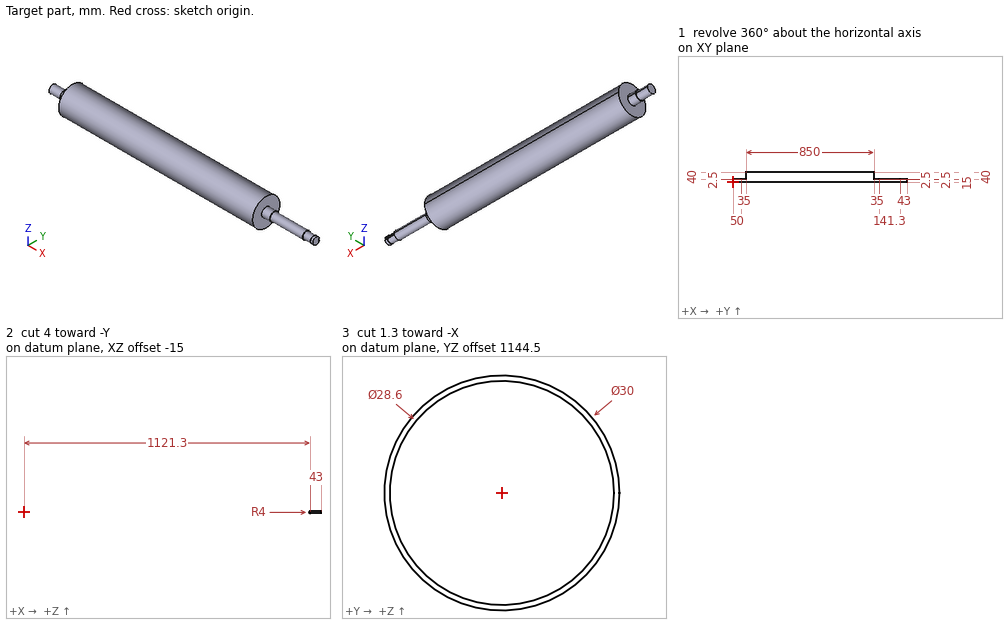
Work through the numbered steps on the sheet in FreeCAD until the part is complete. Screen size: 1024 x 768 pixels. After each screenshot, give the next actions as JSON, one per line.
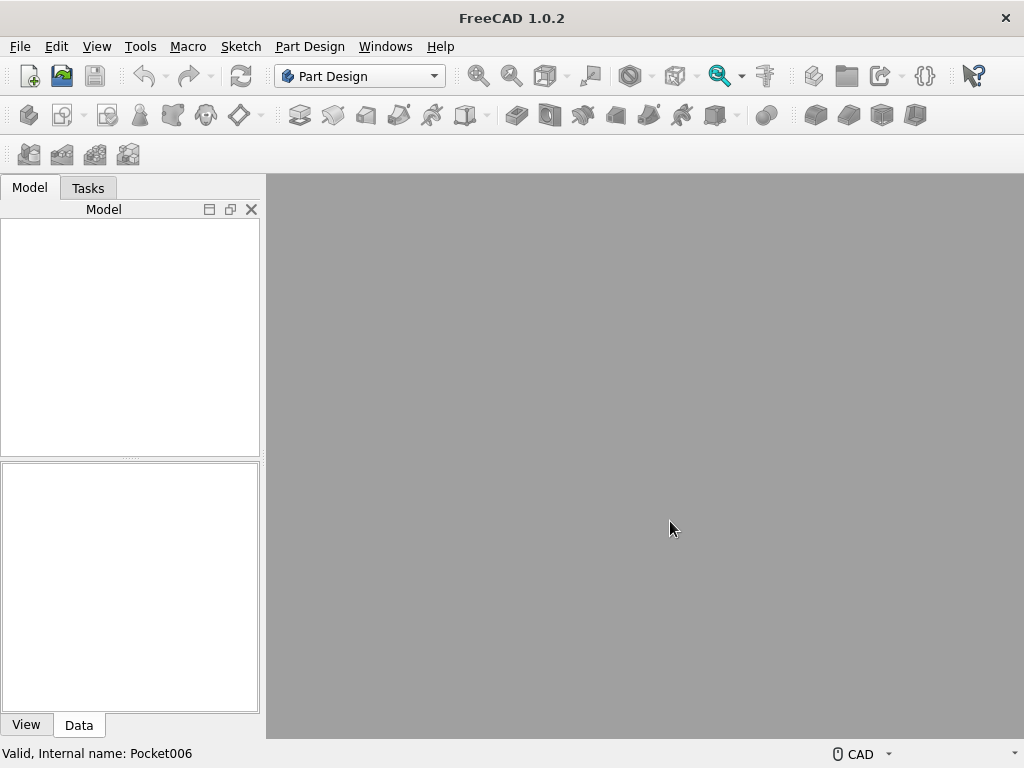
{"action": "key", "text": "ctrl+n"}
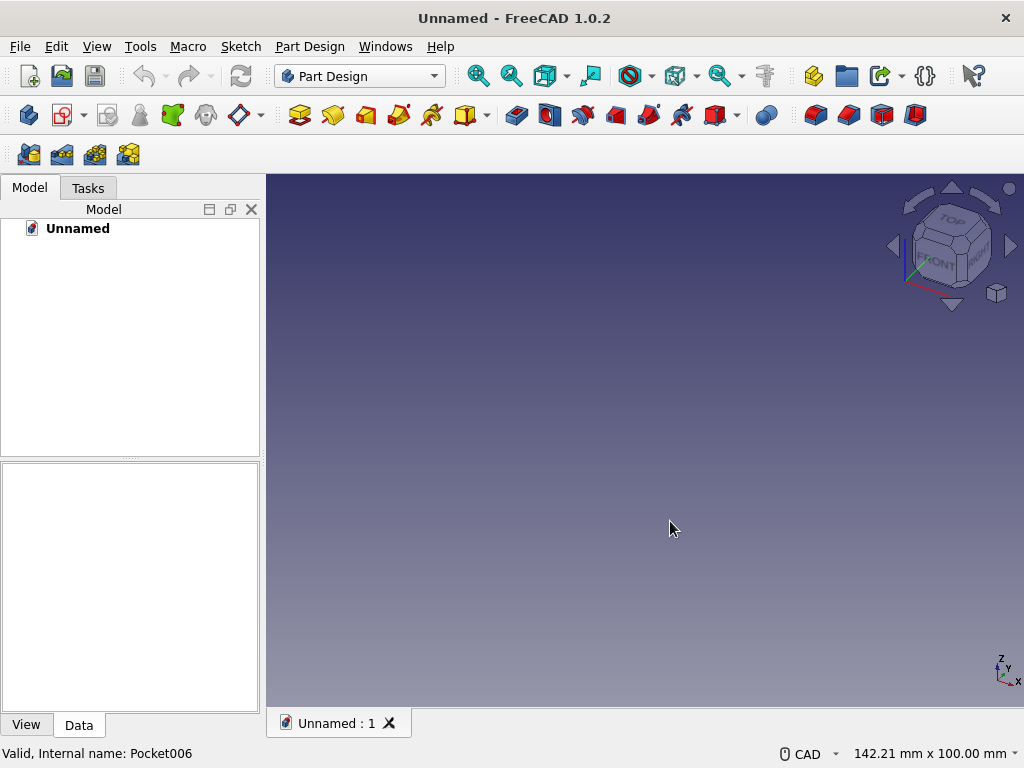
{"action": "left_click", "coordinate": [62, 116]}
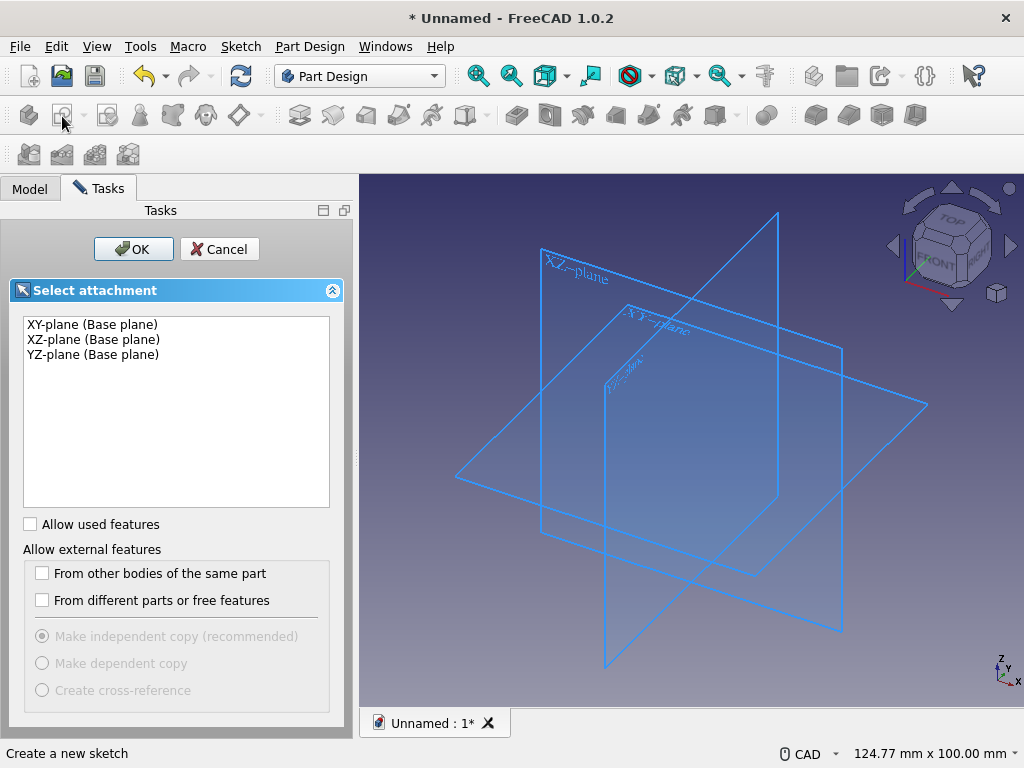
{"action": "left_click", "coordinate": [84, 324]}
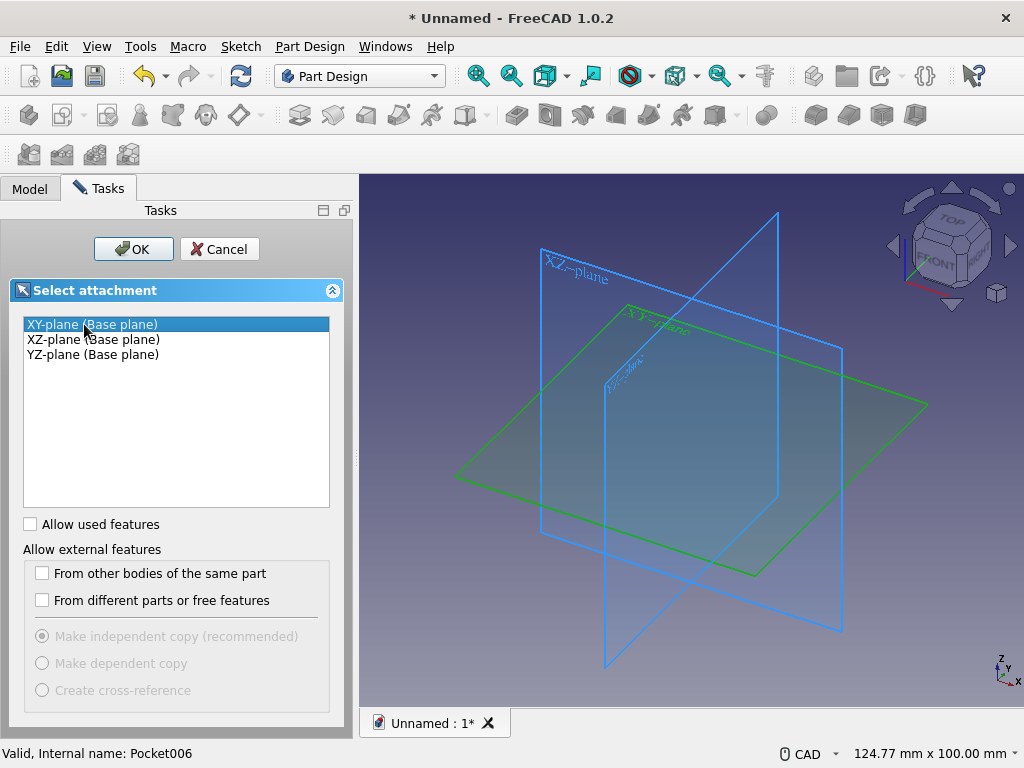
{"action": "left_click", "coordinate": [134, 249]}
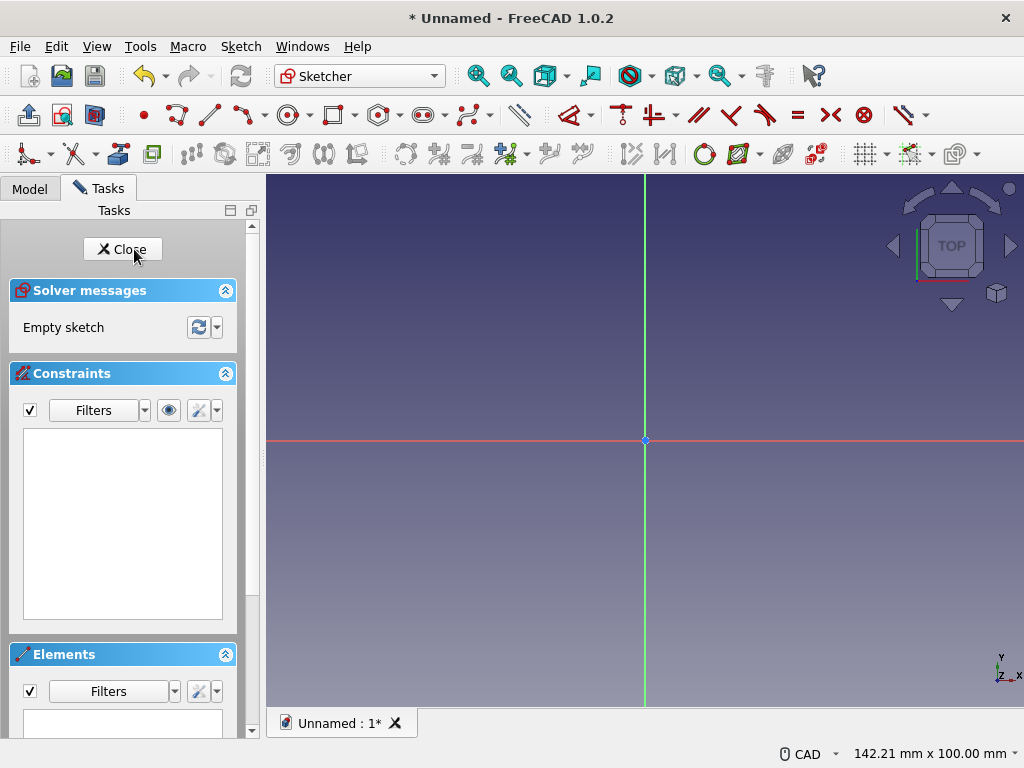
{"action": "scroll", "coordinate": [373, 451], "scroll_direction": "down", "scroll_amount": 14}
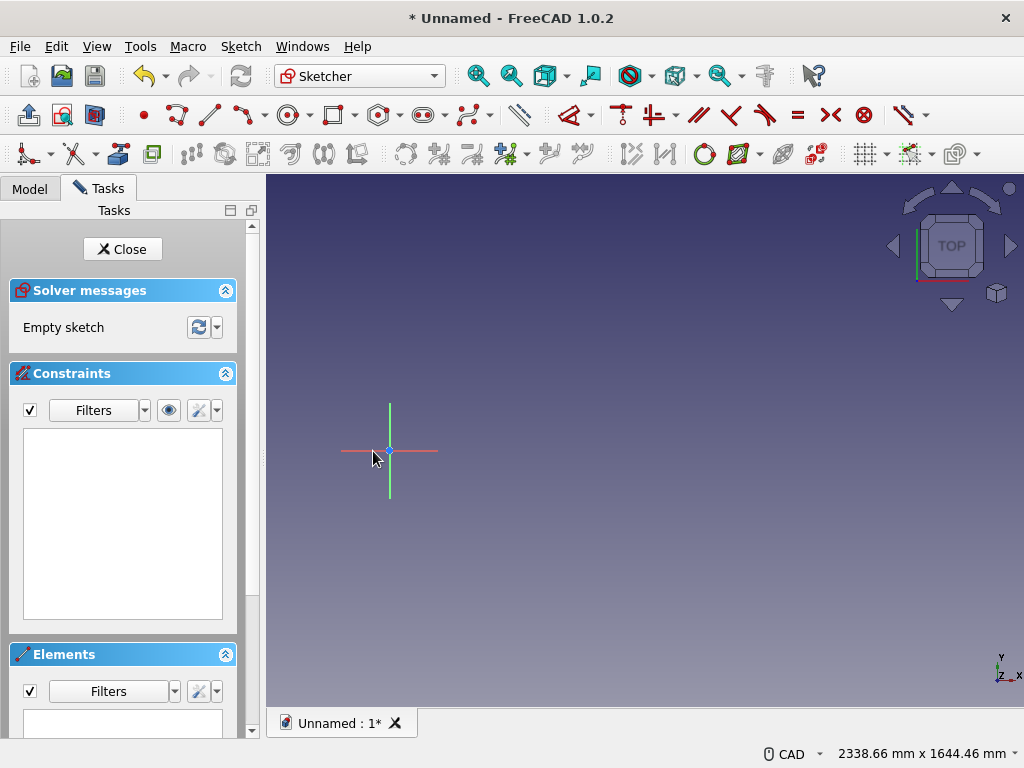
{"action": "key", "text": "g m"}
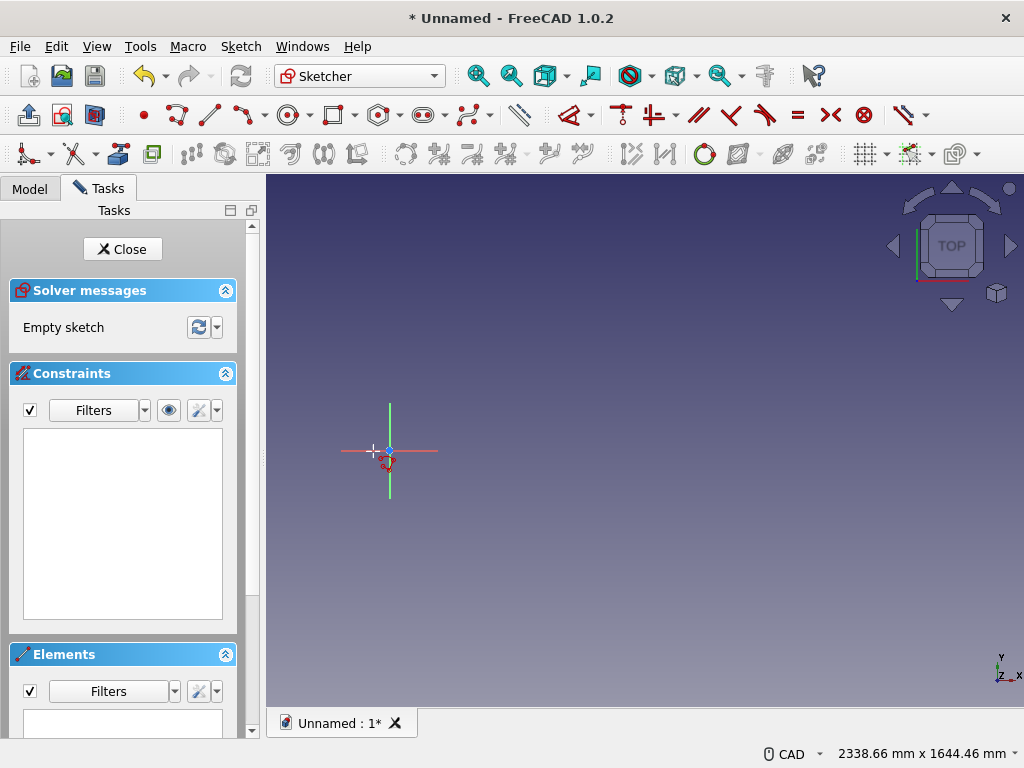
{"action": "left_click", "coordinate": [390, 451]}
{"action": "left_click", "coordinate": [764, 442]}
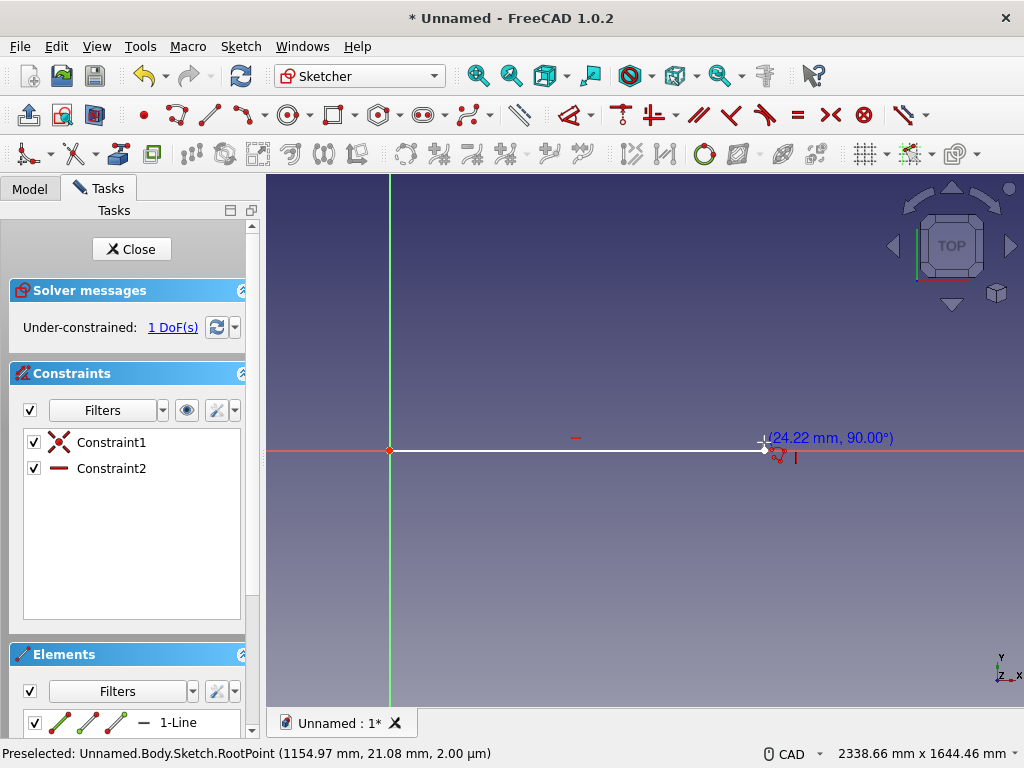
{"action": "scroll", "coordinate": [764, 446], "scroll_direction": "up", "scroll_amount": 6}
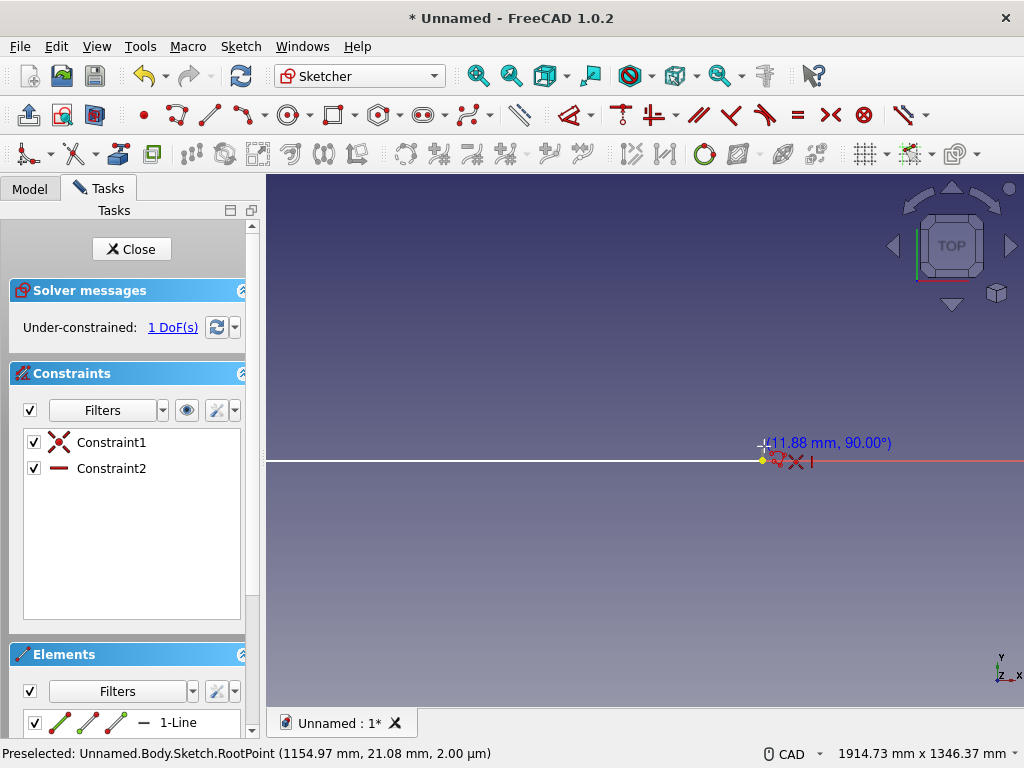
{"action": "left_click", "coordinate": [762, 445]}
{"action": "left_click", "coordinate": [716, 445]}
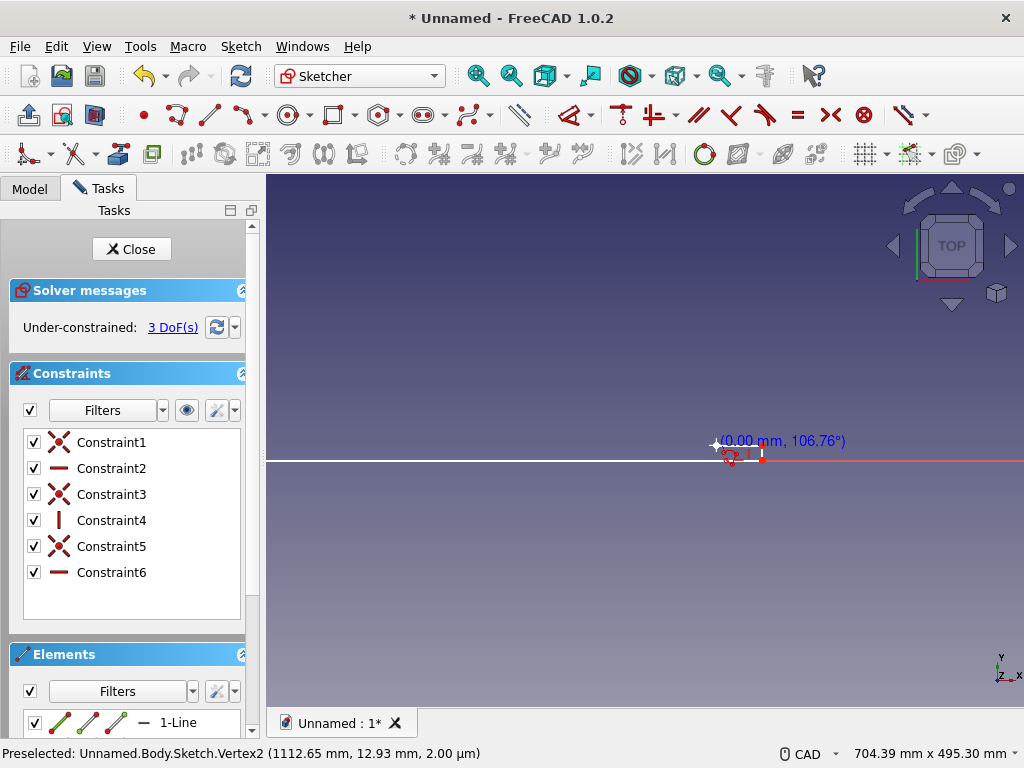
{"action": "scroll", "coordinate": [716, 442], "scroll_direction": "up", "scroll_amount": 9}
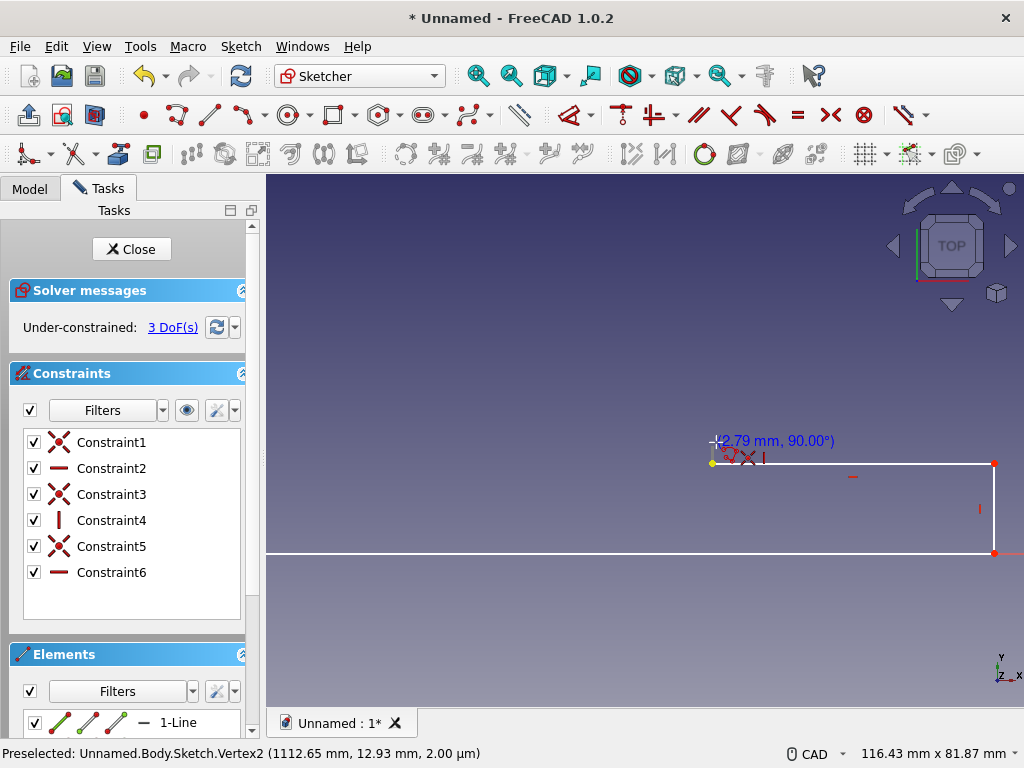
{"action": "left_click", "coordinate": [713, 440]}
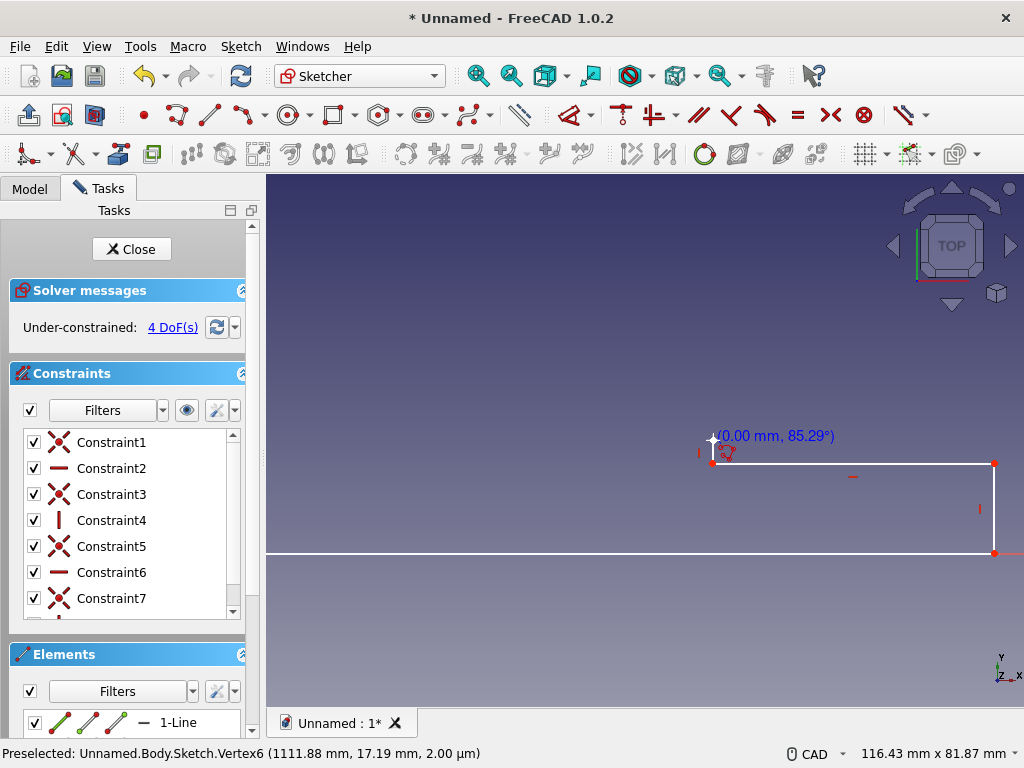
{"action": "scroll", "coordinate": [752, 445], "scroll_direction": "down", "scroll_amount": 15}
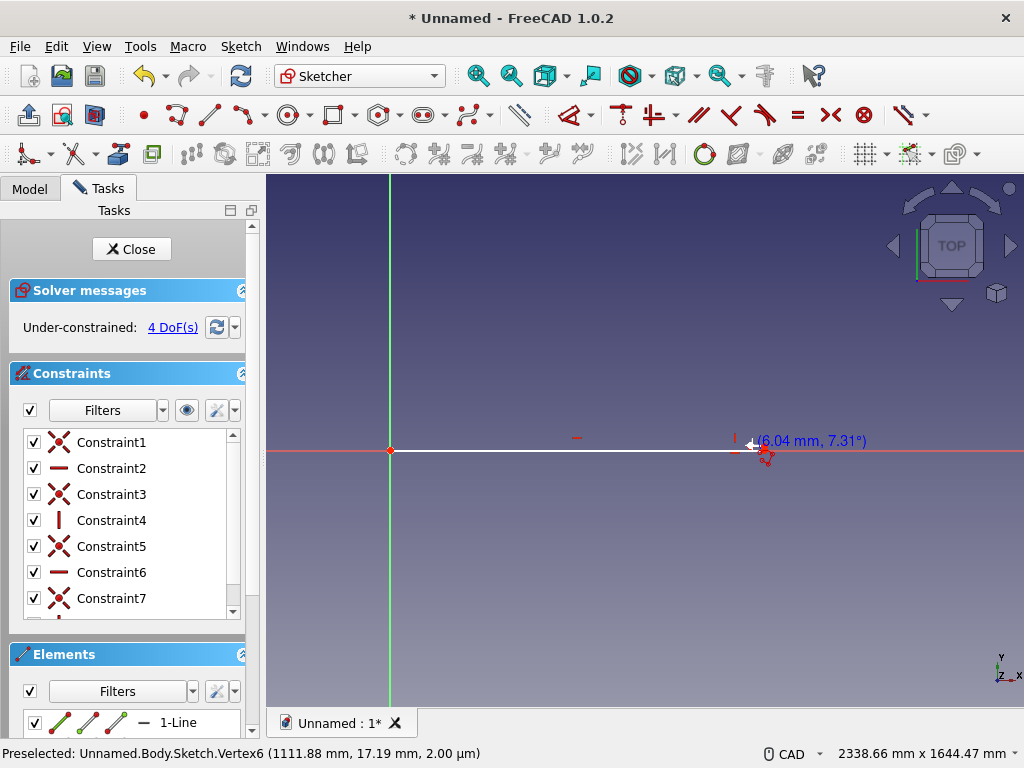
{"action": "scroll", "coordinate": [705, 445], "scroll_direction": "up", "scroll_amount": 6}